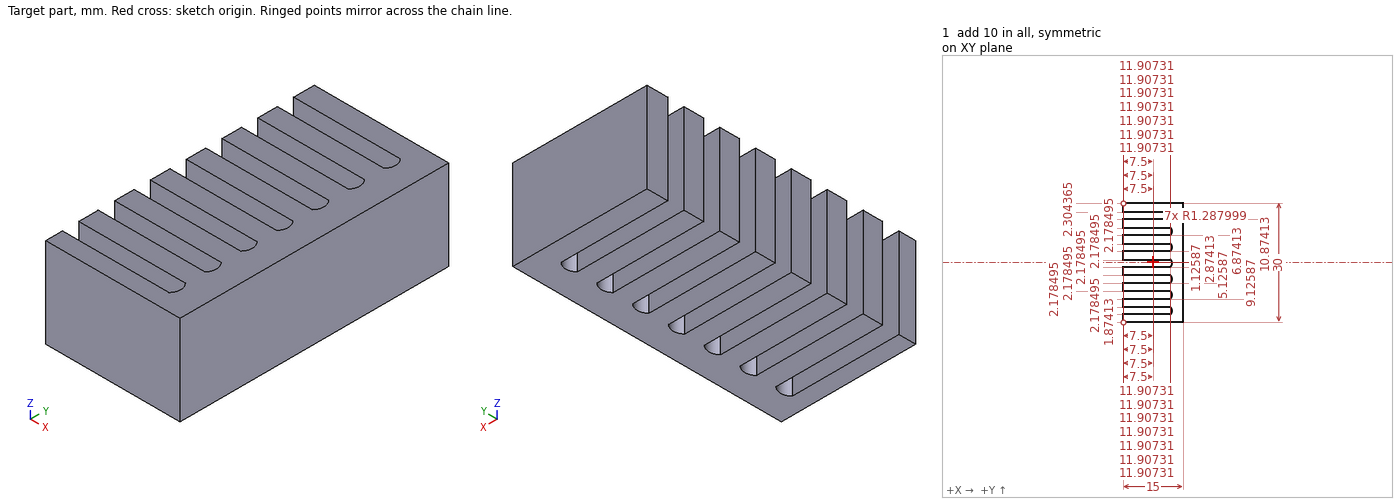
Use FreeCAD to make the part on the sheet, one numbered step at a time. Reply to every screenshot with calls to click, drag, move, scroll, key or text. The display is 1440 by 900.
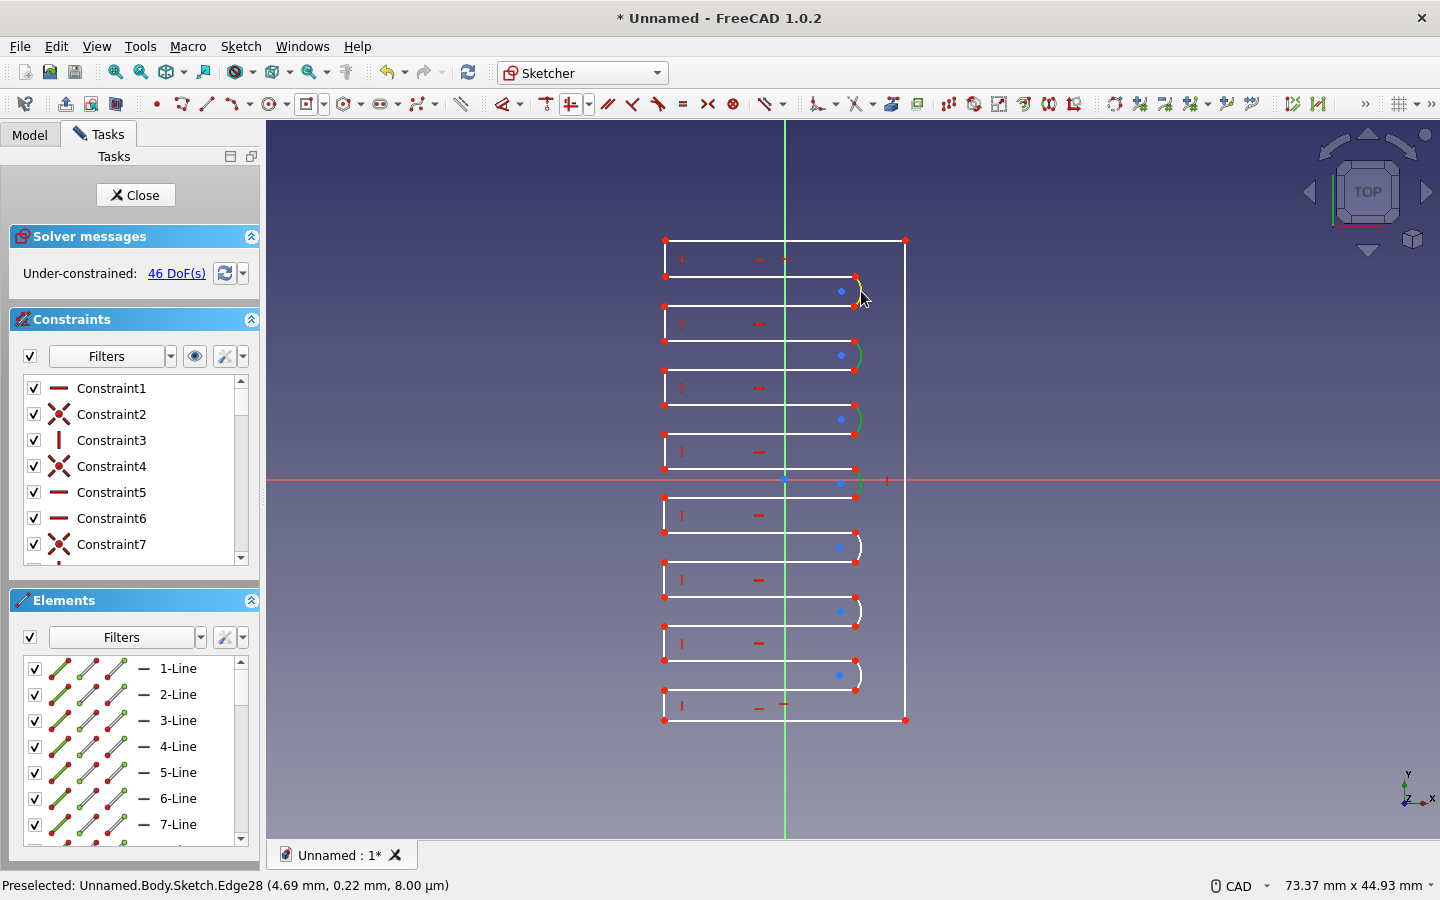
scroll(860, 554, up, 2)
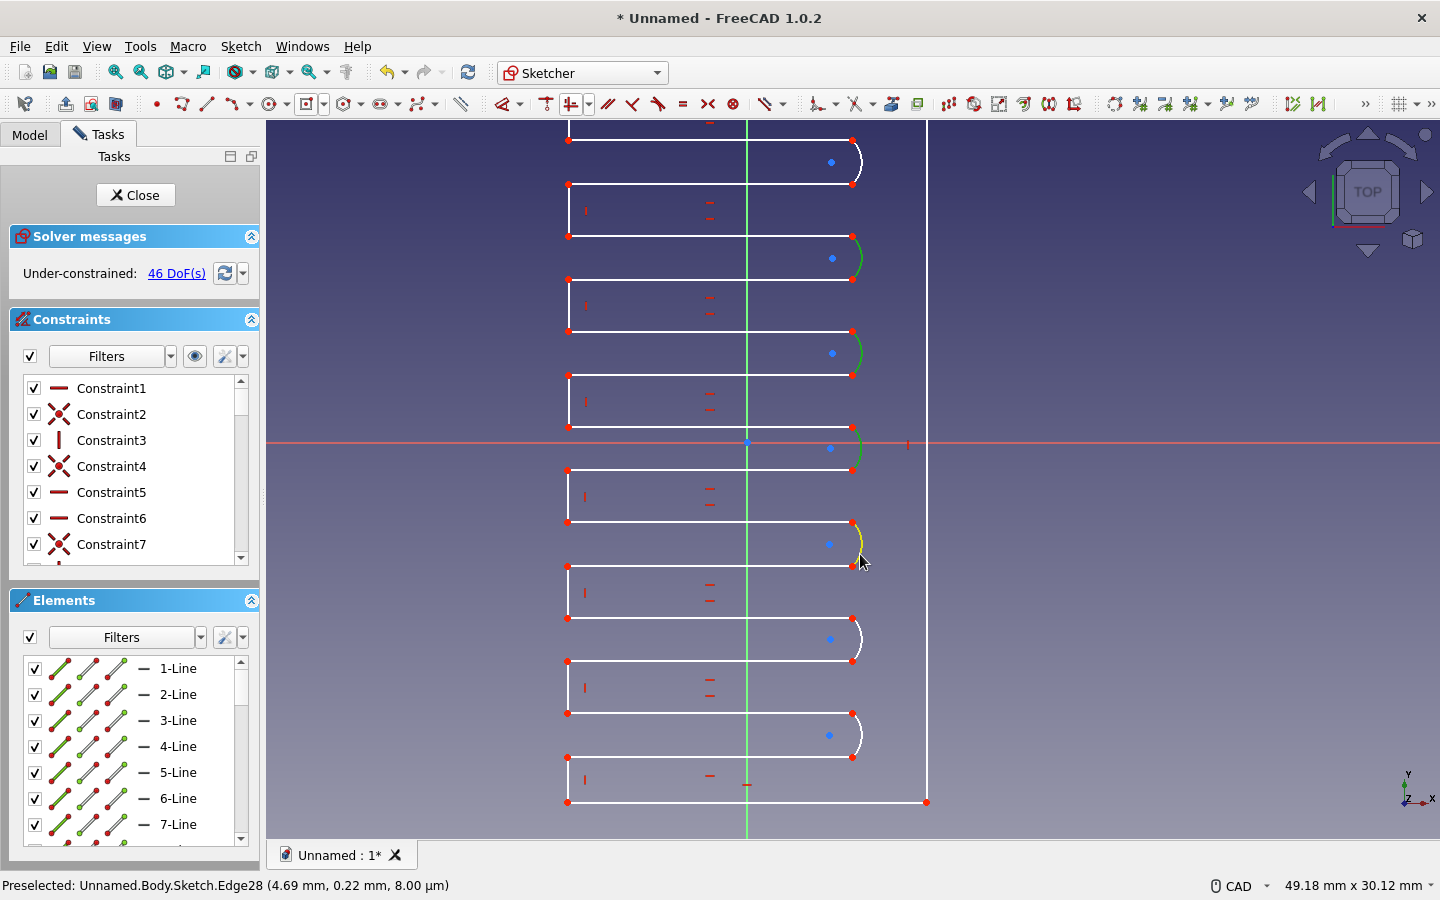
click(860, 554)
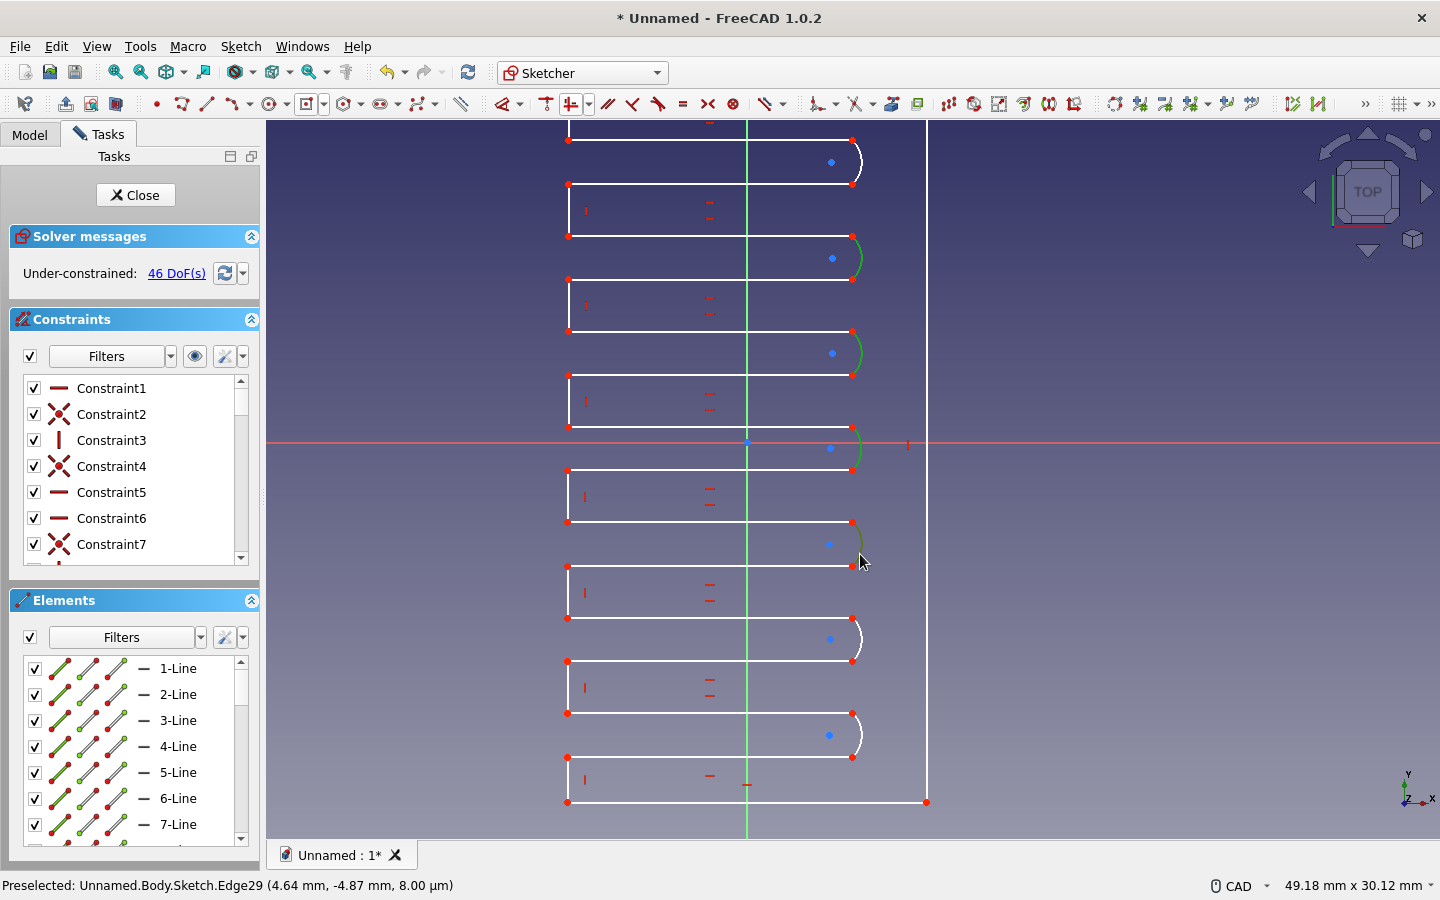
click(860, 649)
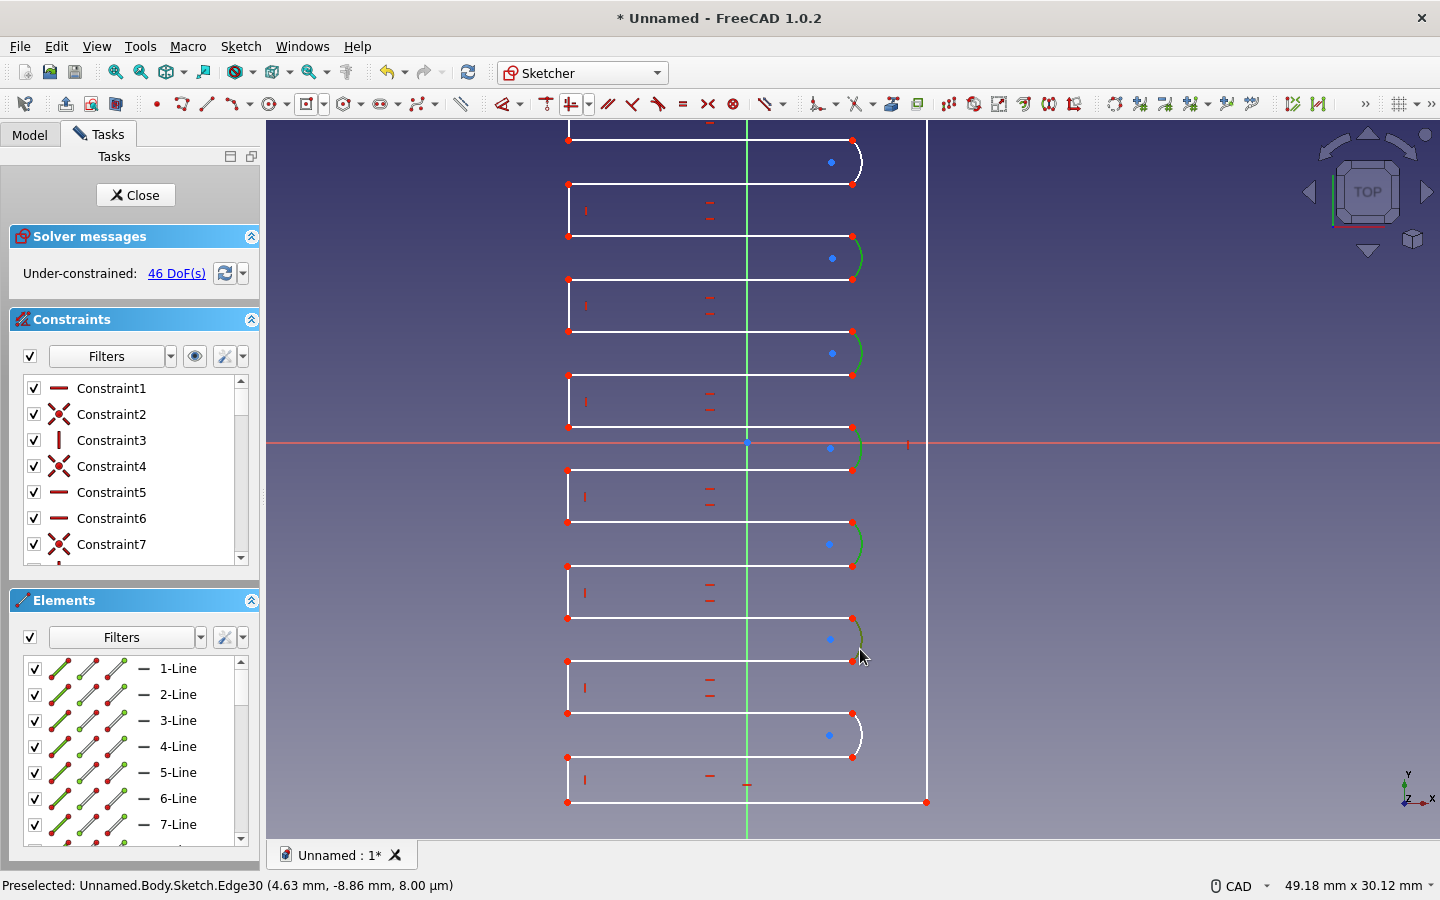
click(860, 745)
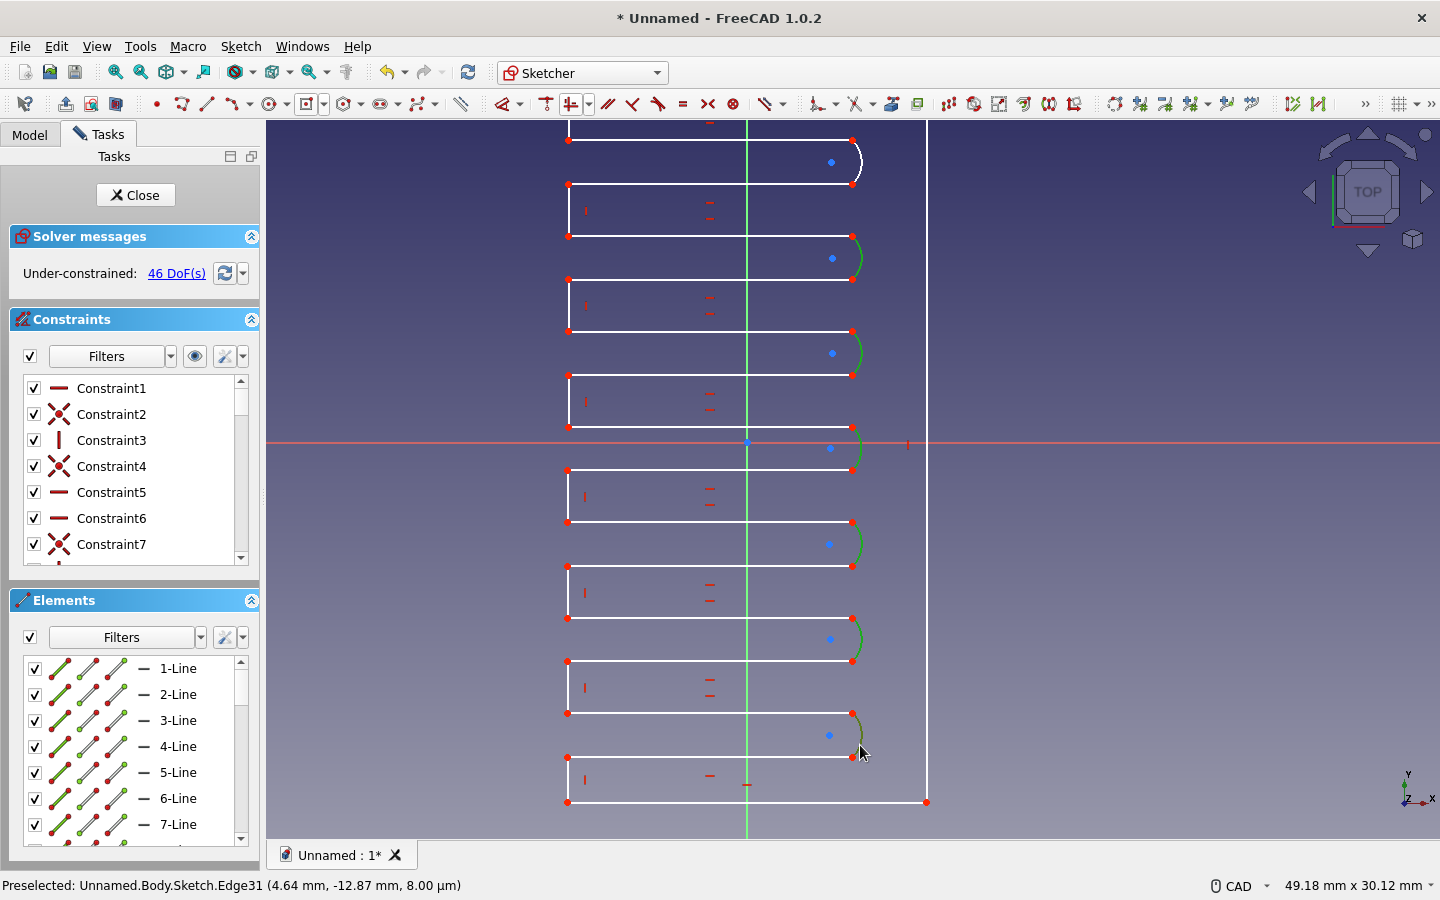
click(860, 172)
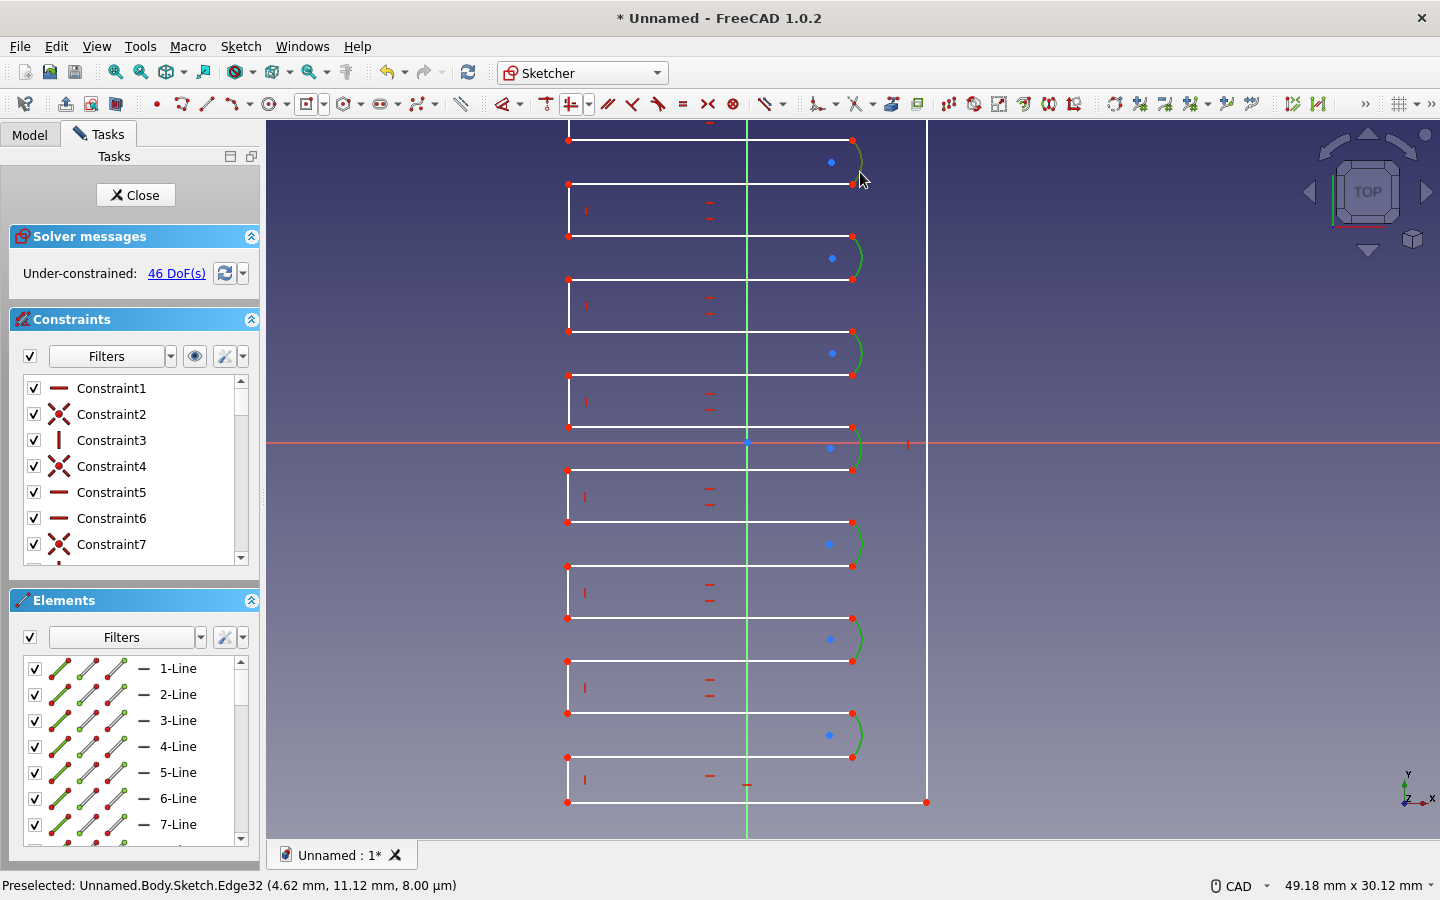
click(683, 104)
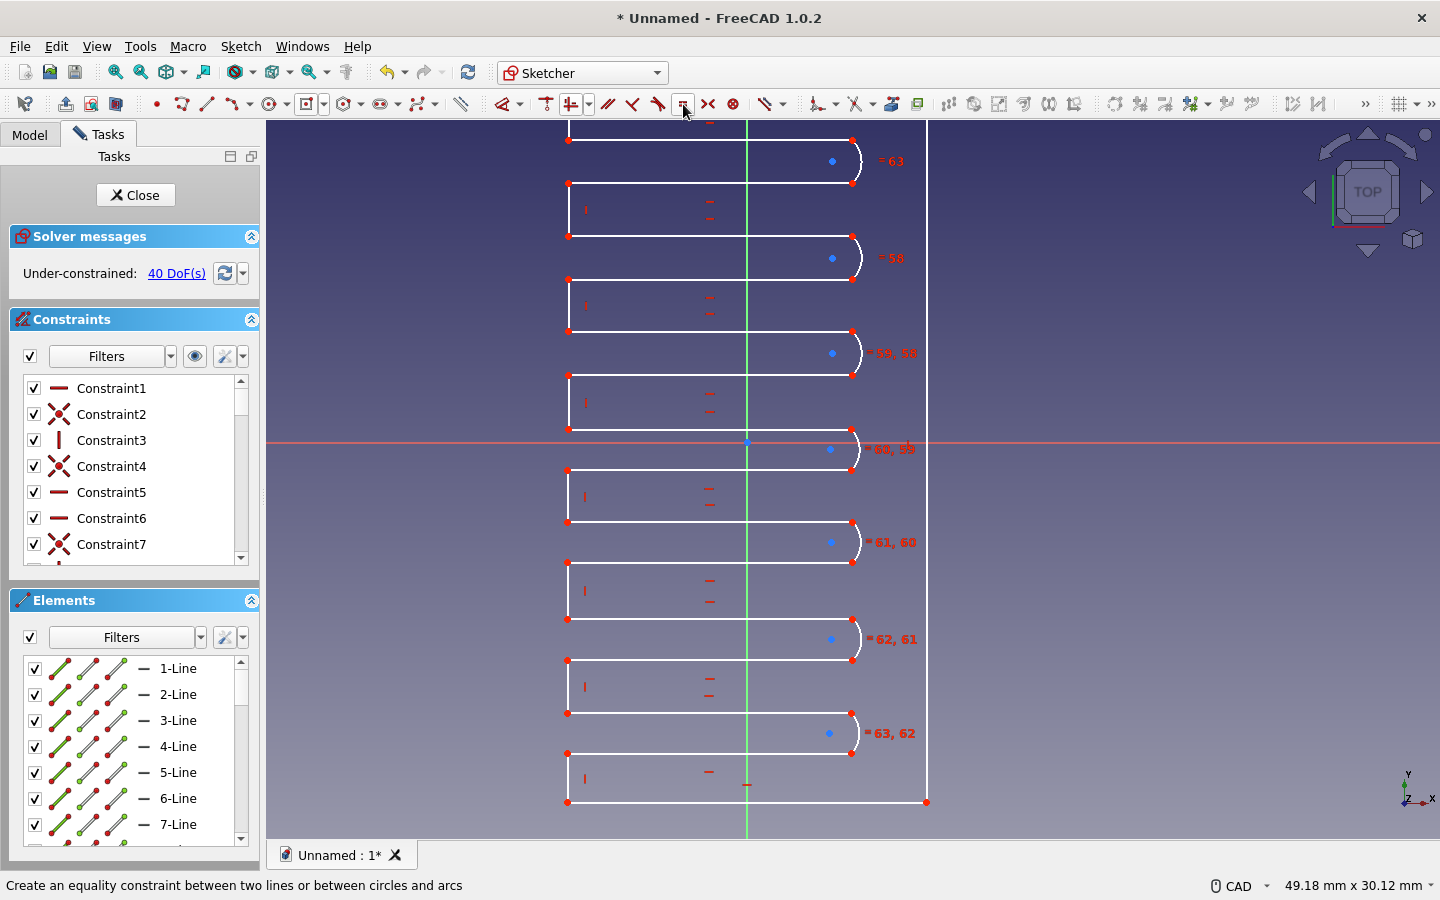
click(568, 803)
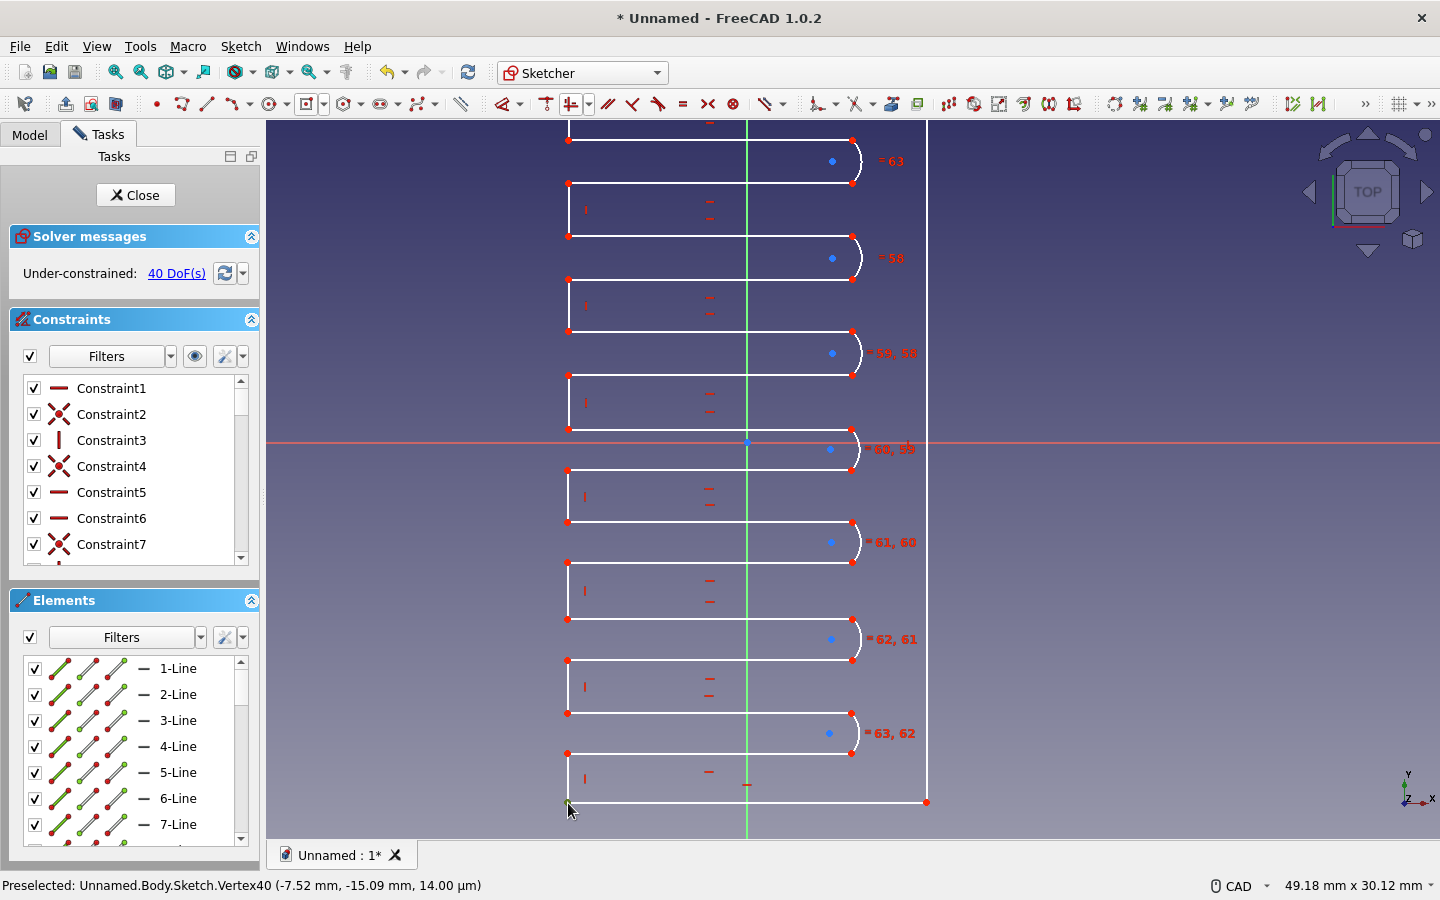
scroll(860, 554, down, 2)